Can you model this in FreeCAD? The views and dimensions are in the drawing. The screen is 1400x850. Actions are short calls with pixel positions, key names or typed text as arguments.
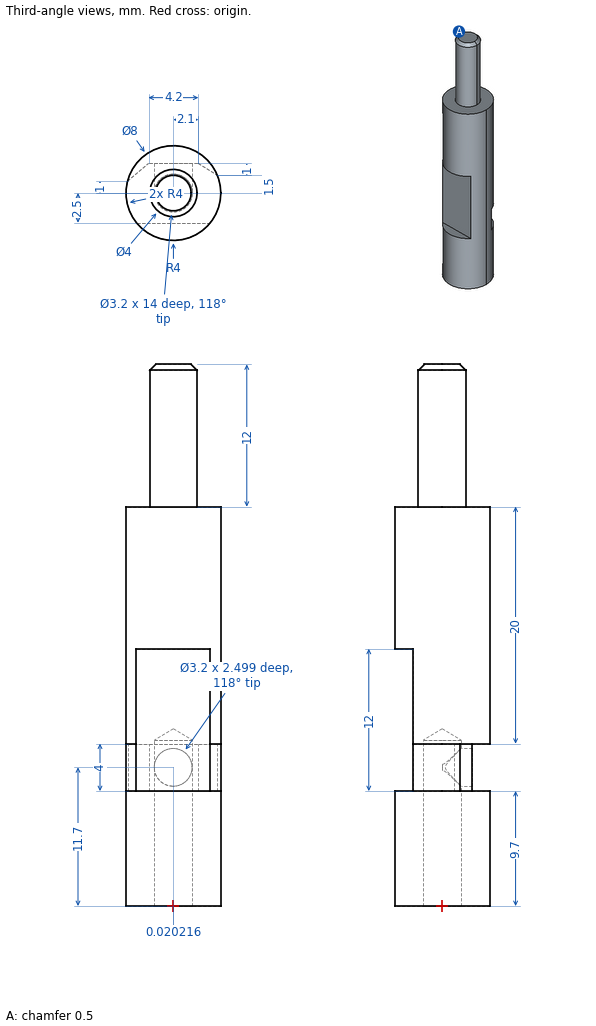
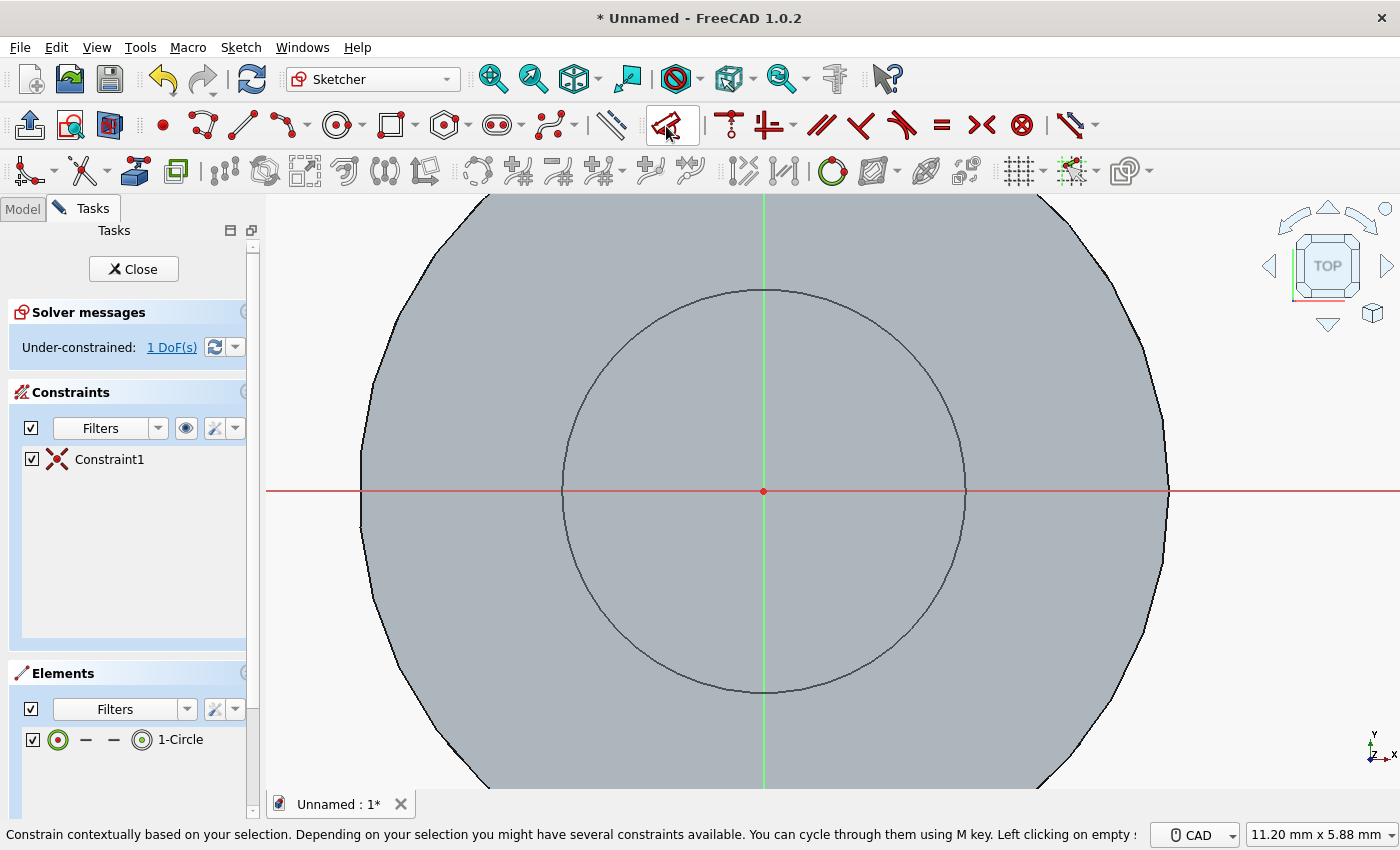
click(906, 348)
click(929, 325)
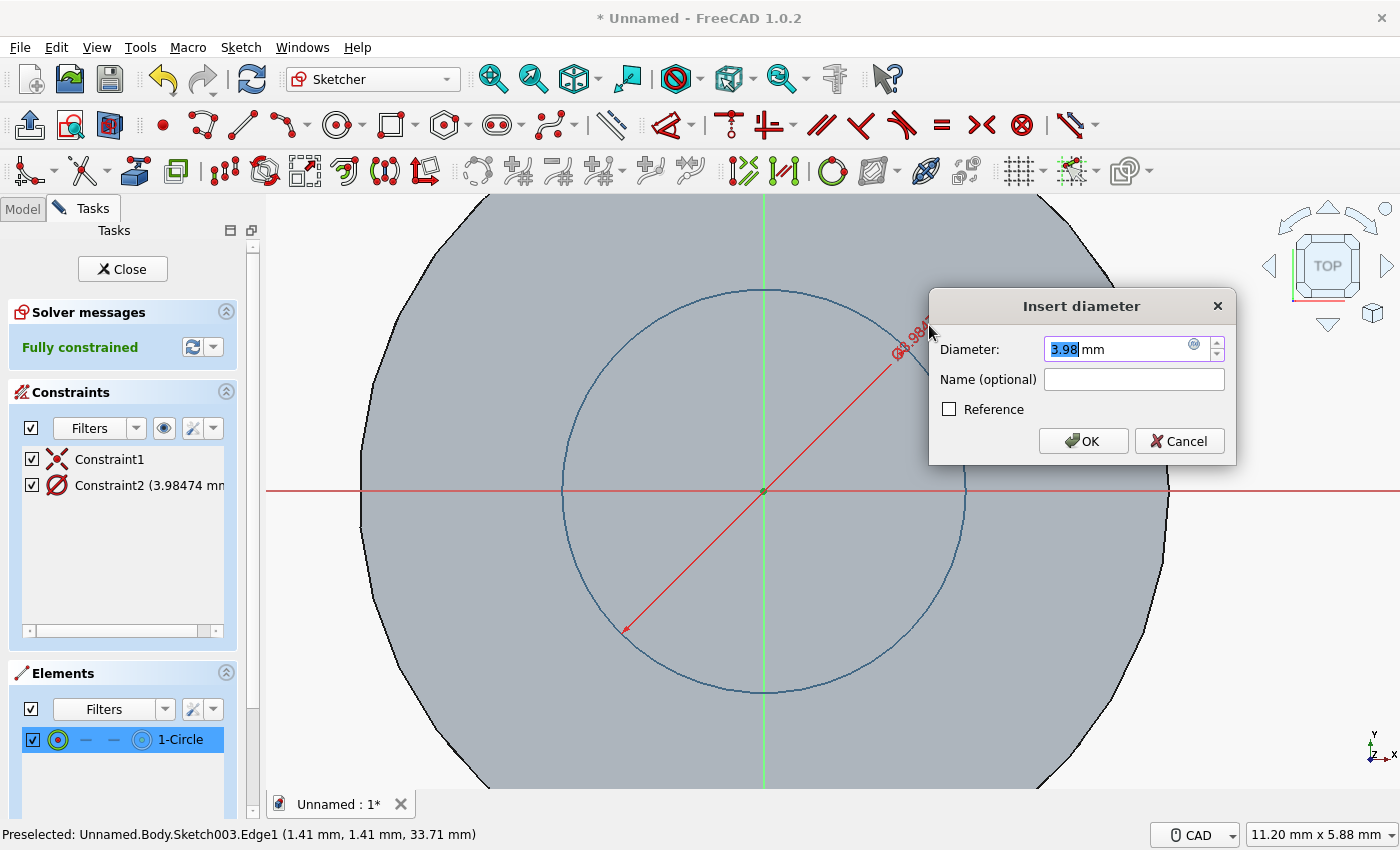
text(4)
key(Return)
key(Escape)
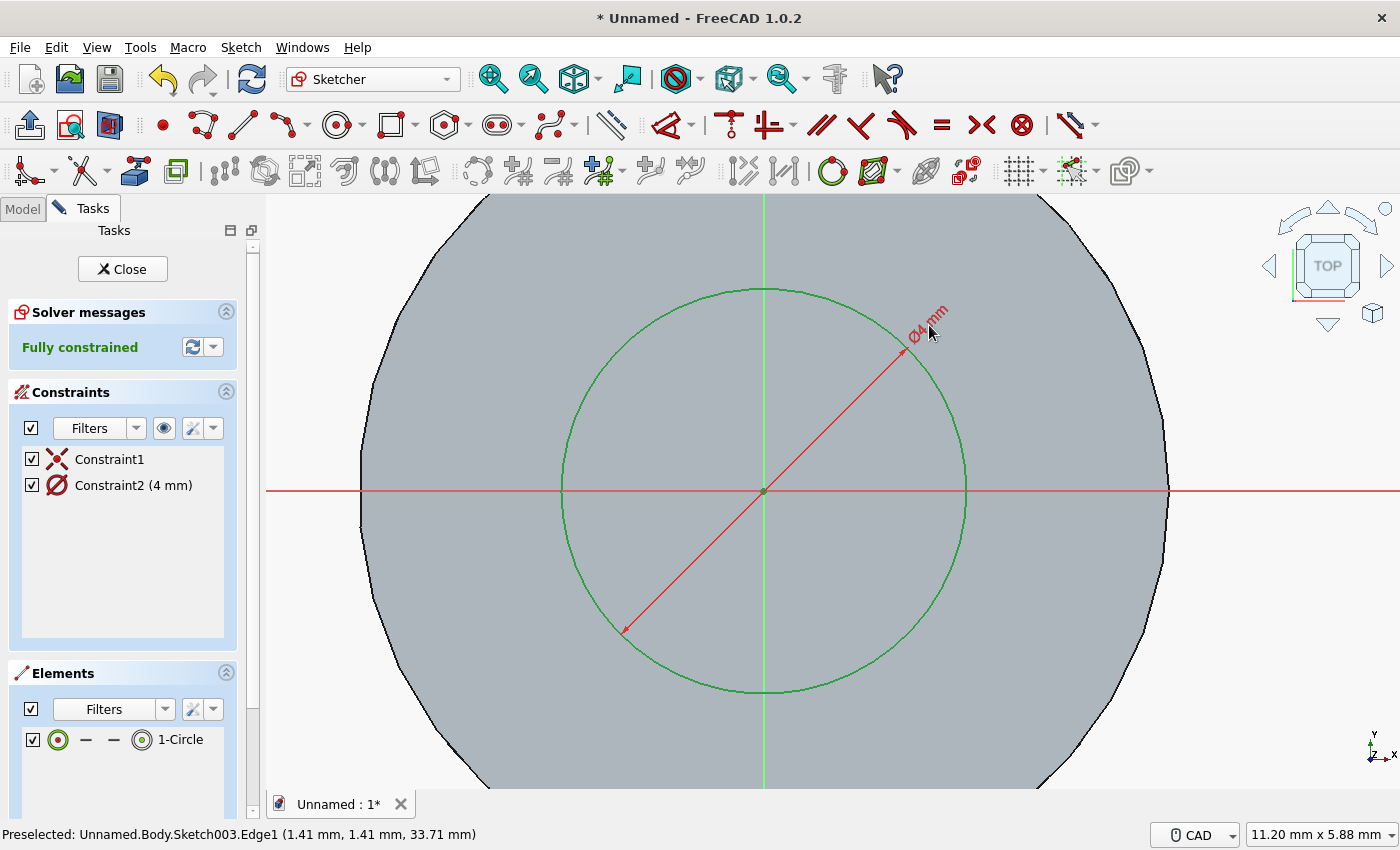
click(123, 269)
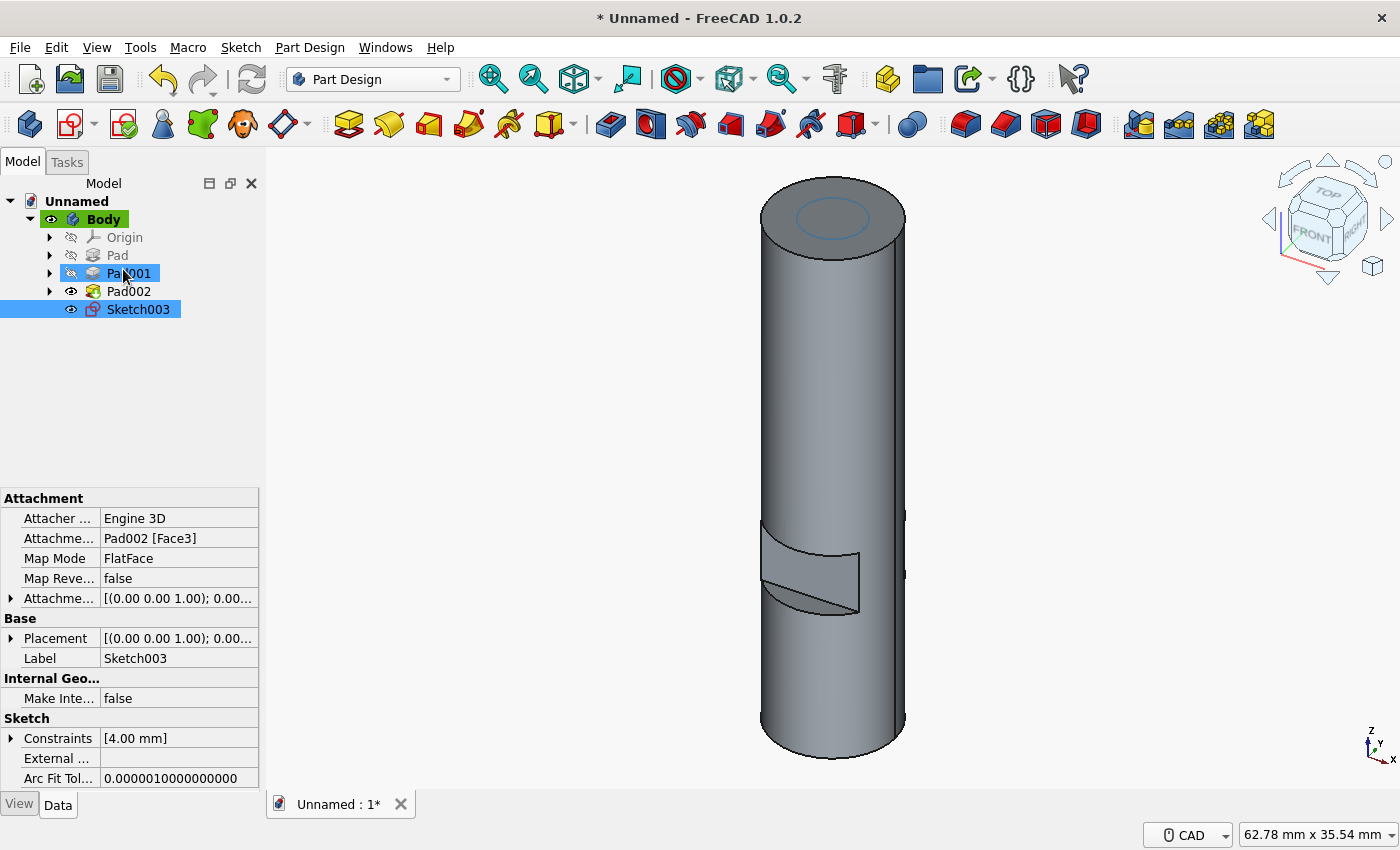
click(350, 124)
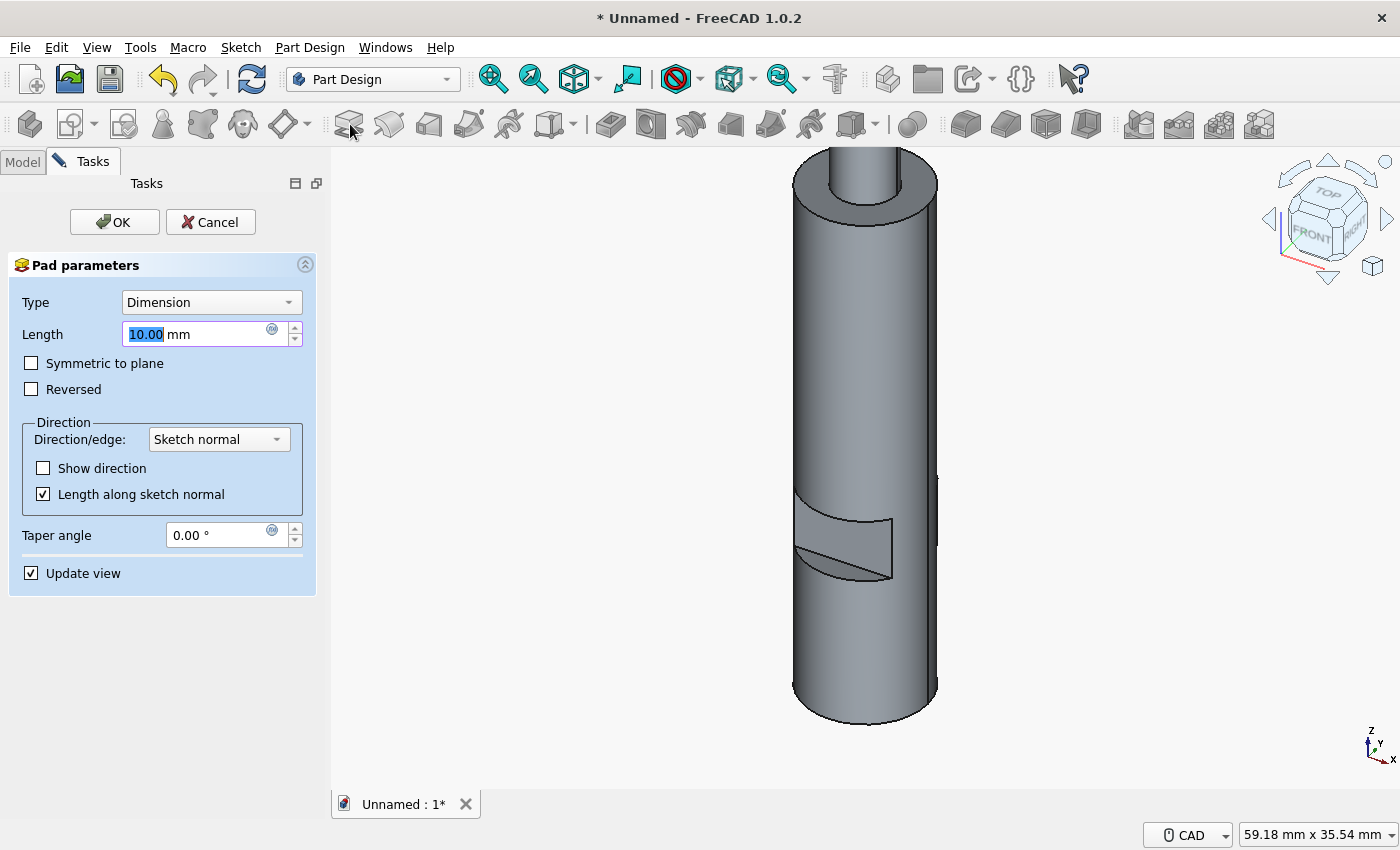
text(12)
key(Tab)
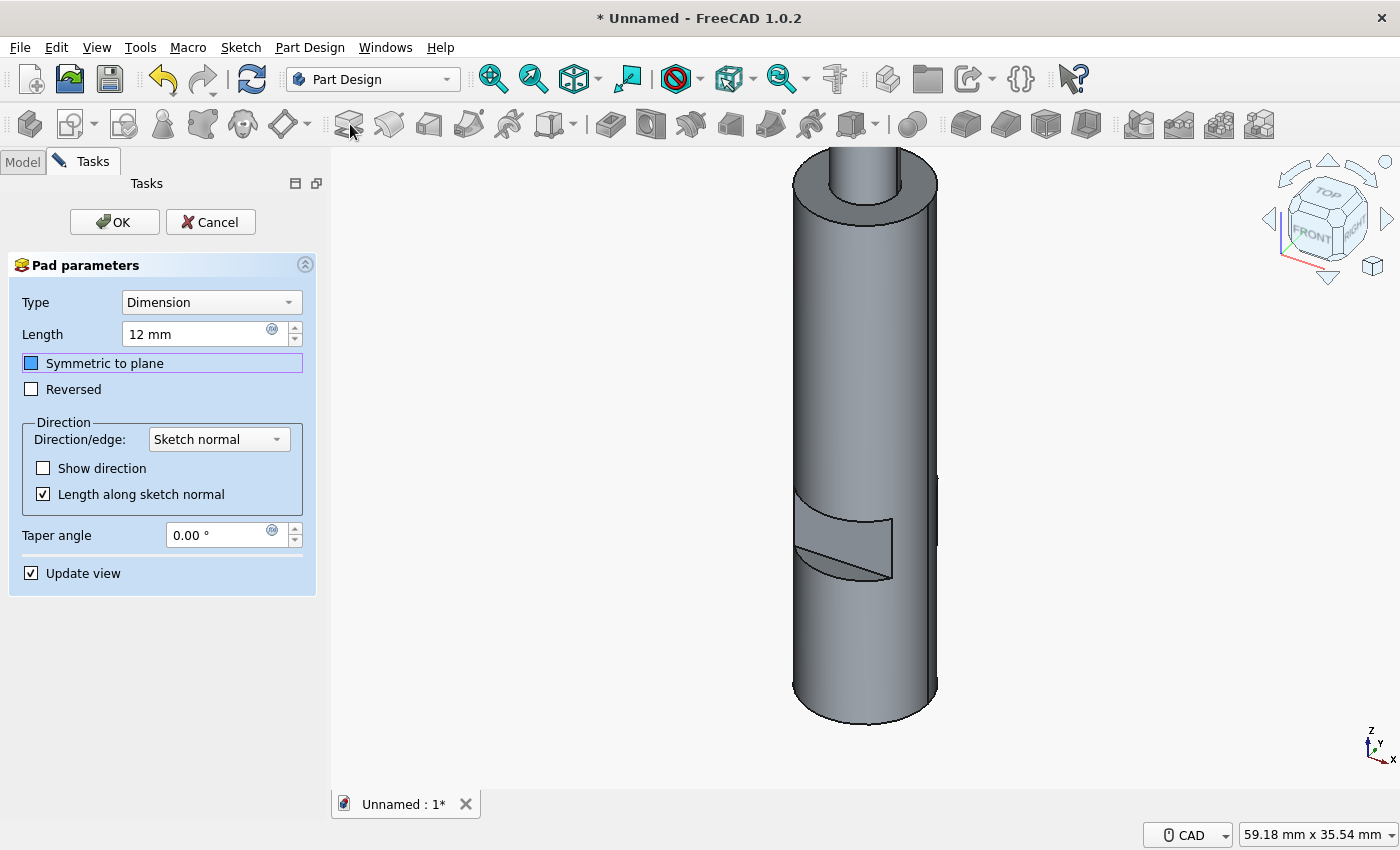
click(115, 222)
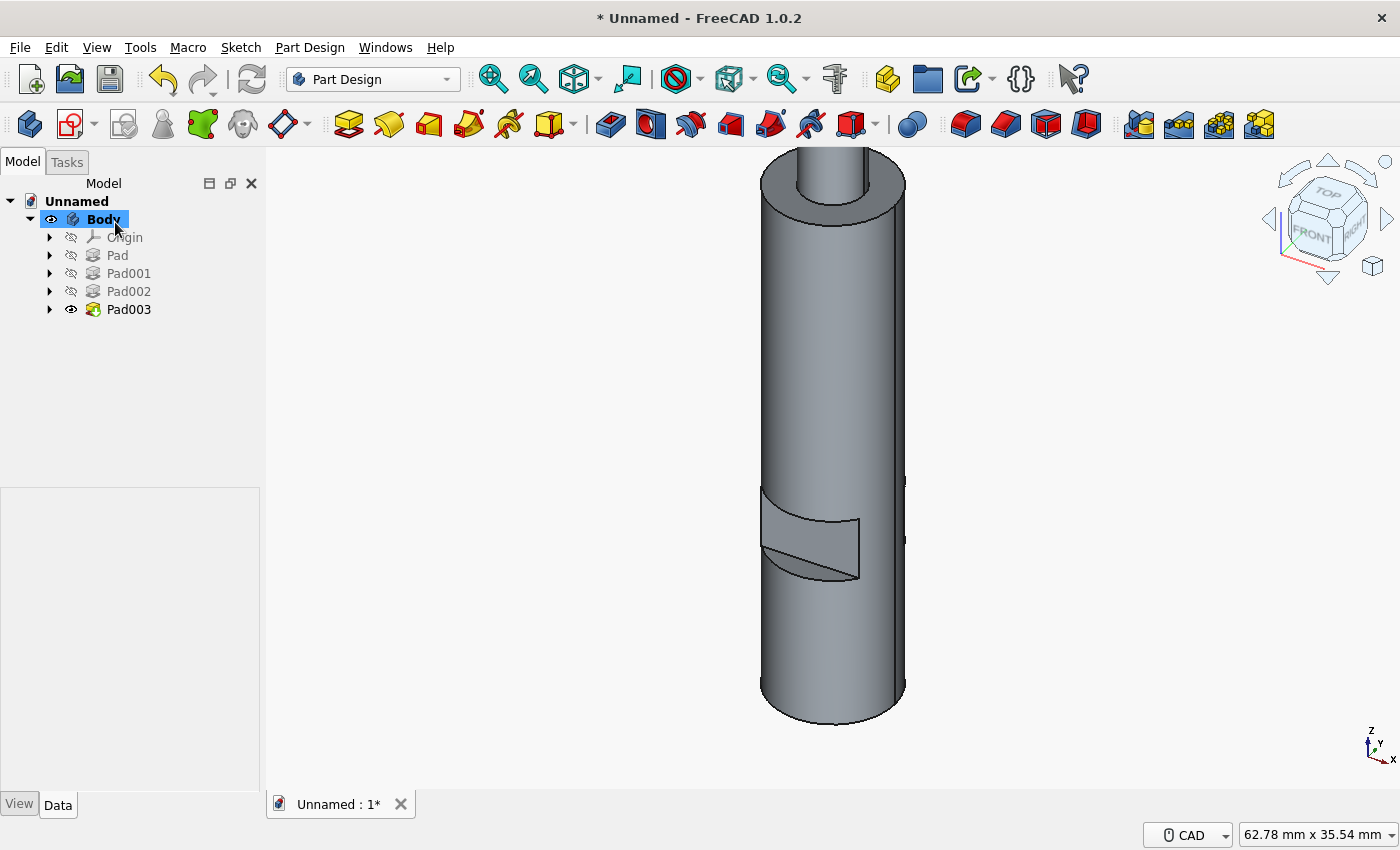
click(494, 80)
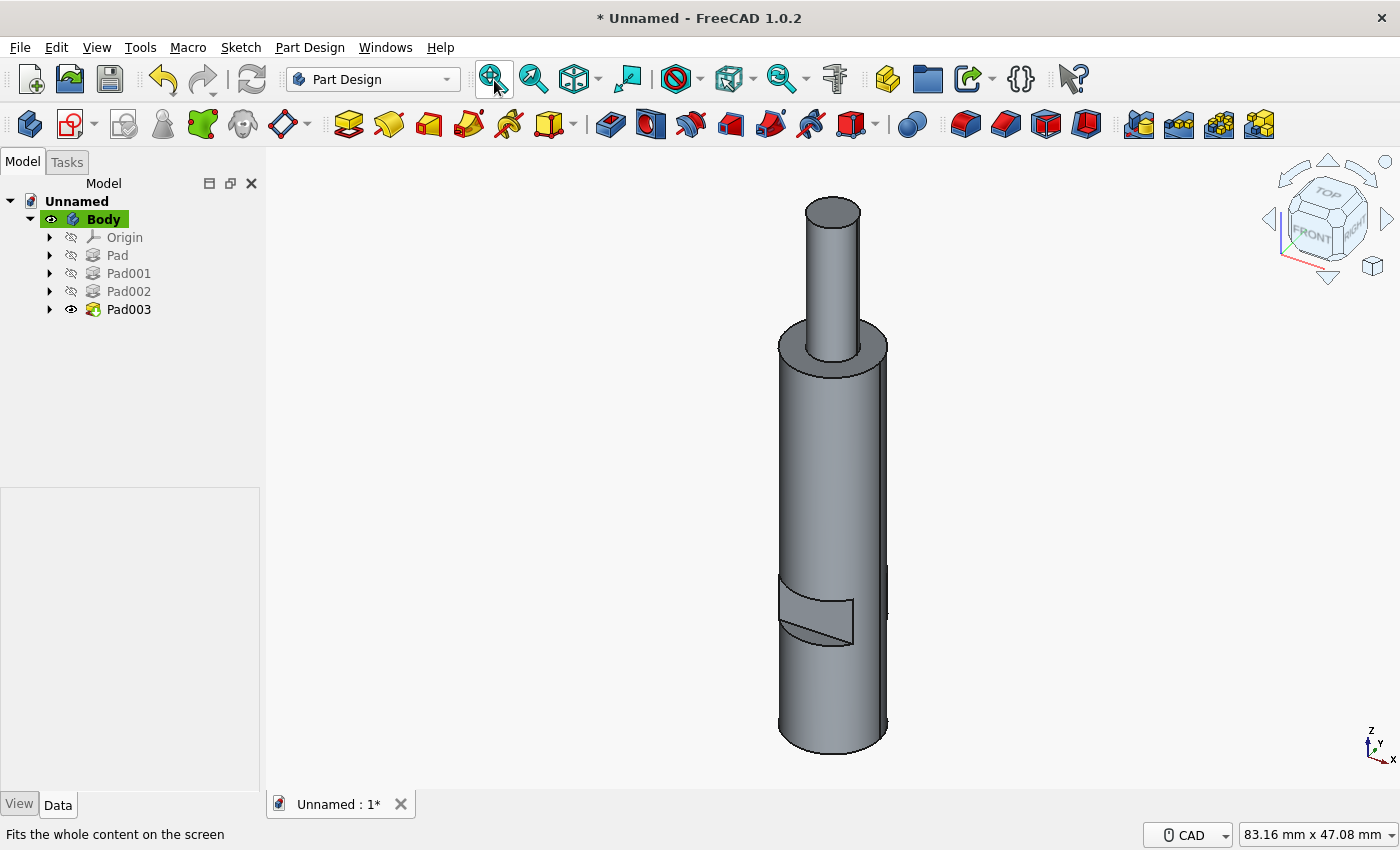
click(806, 213)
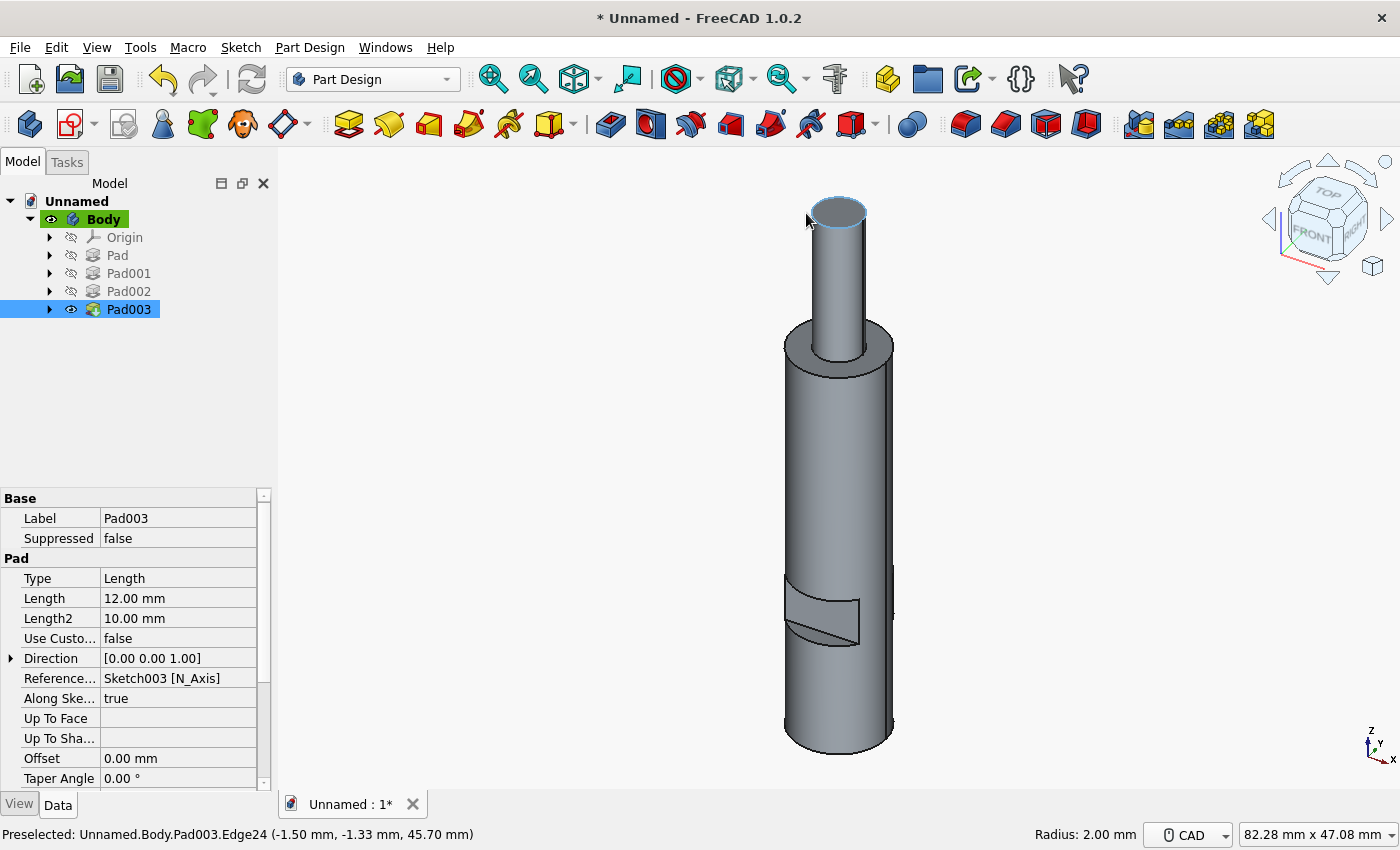
click(1006, 124)